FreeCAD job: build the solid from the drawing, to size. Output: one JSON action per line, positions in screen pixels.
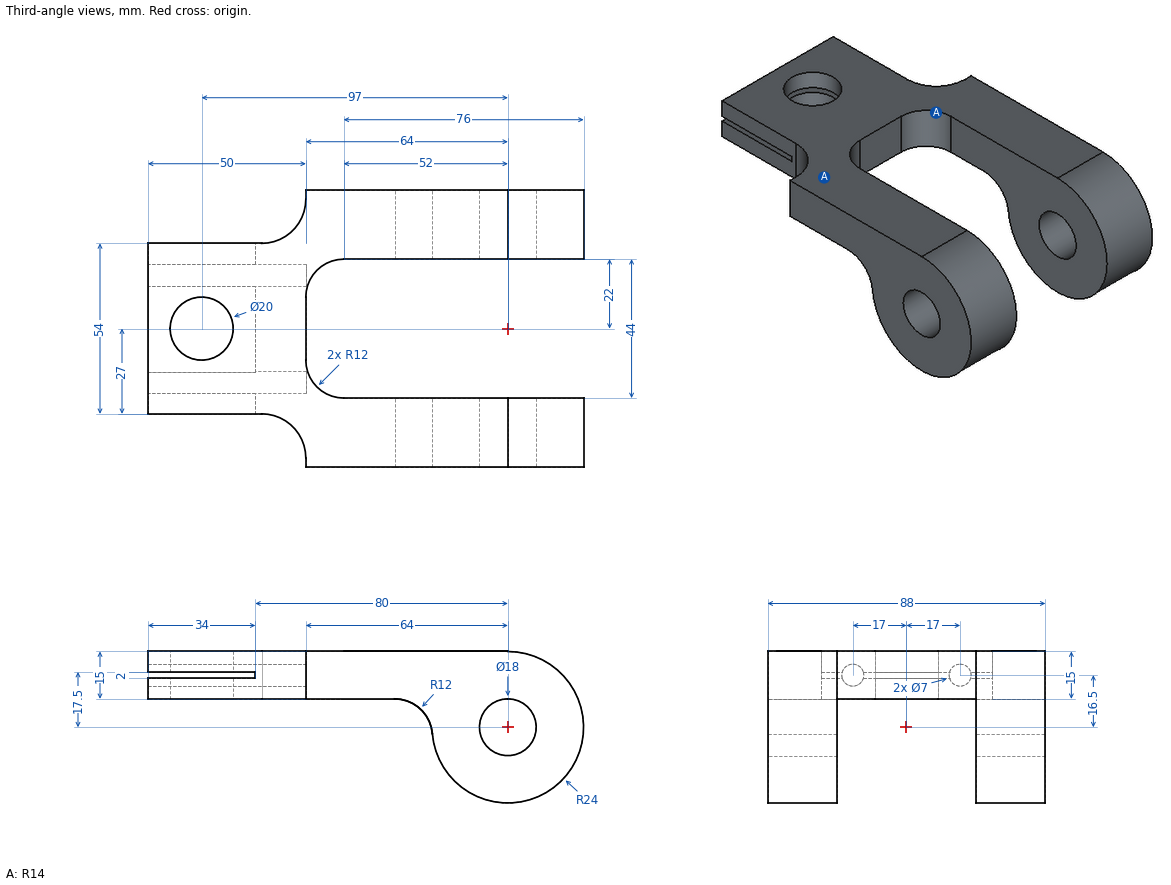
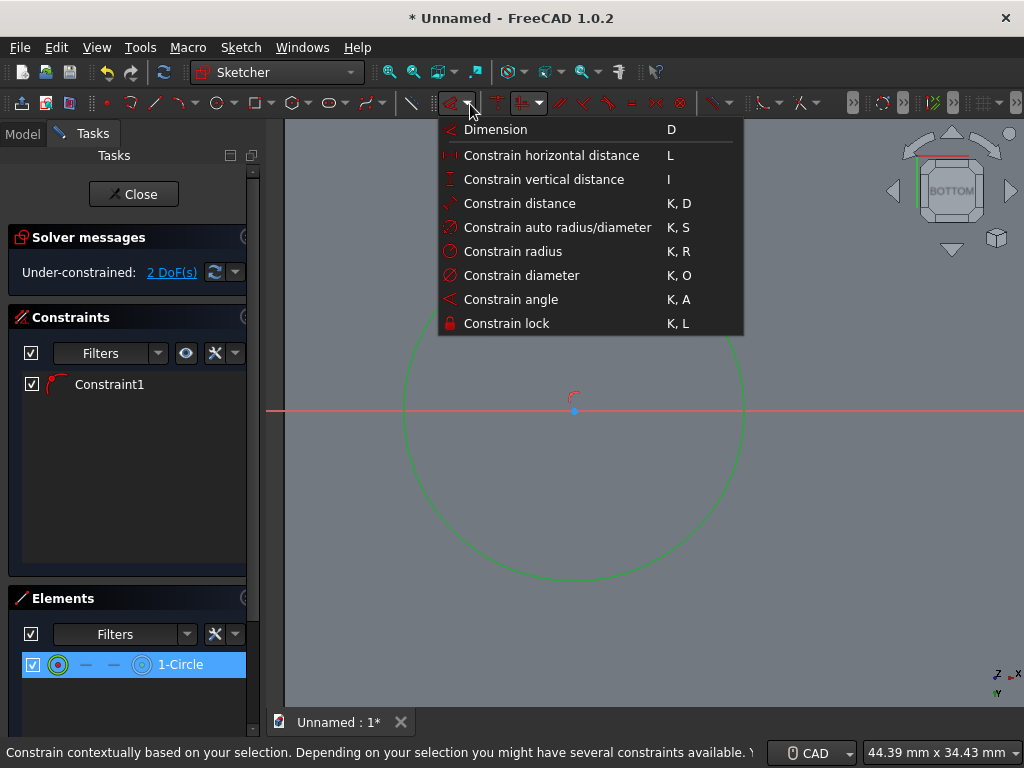
{"action": "left_click", "coordinate": [591, 275]}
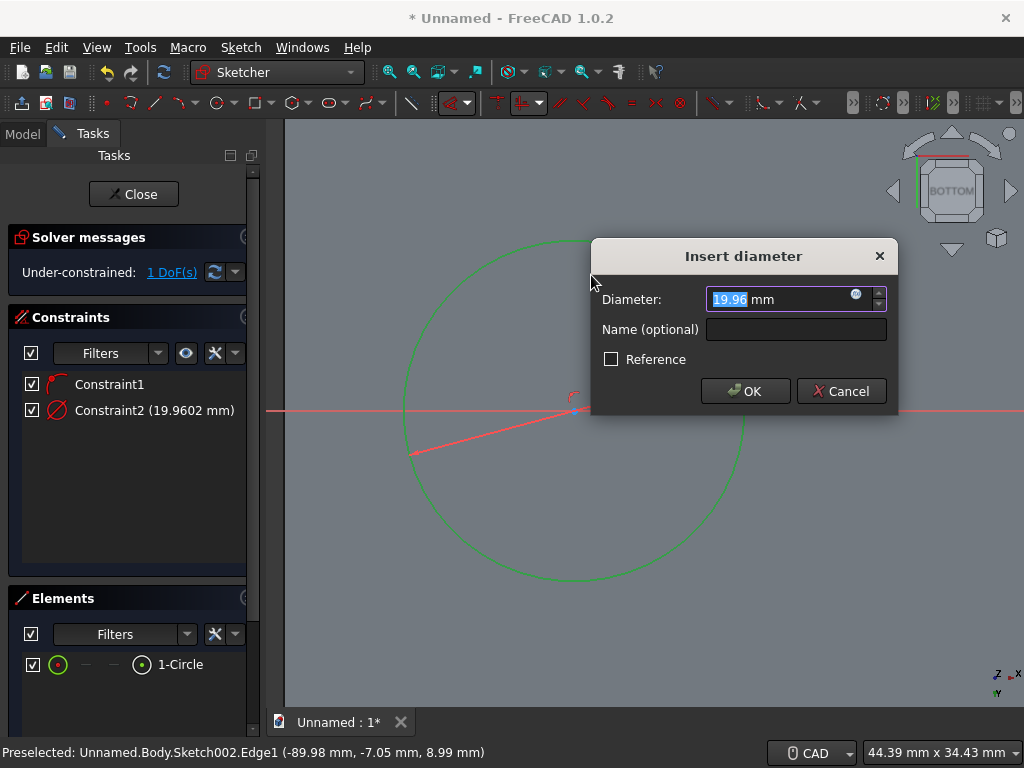
{"action": "type", "text": "20"}
{"action": "key", "text": "Return"}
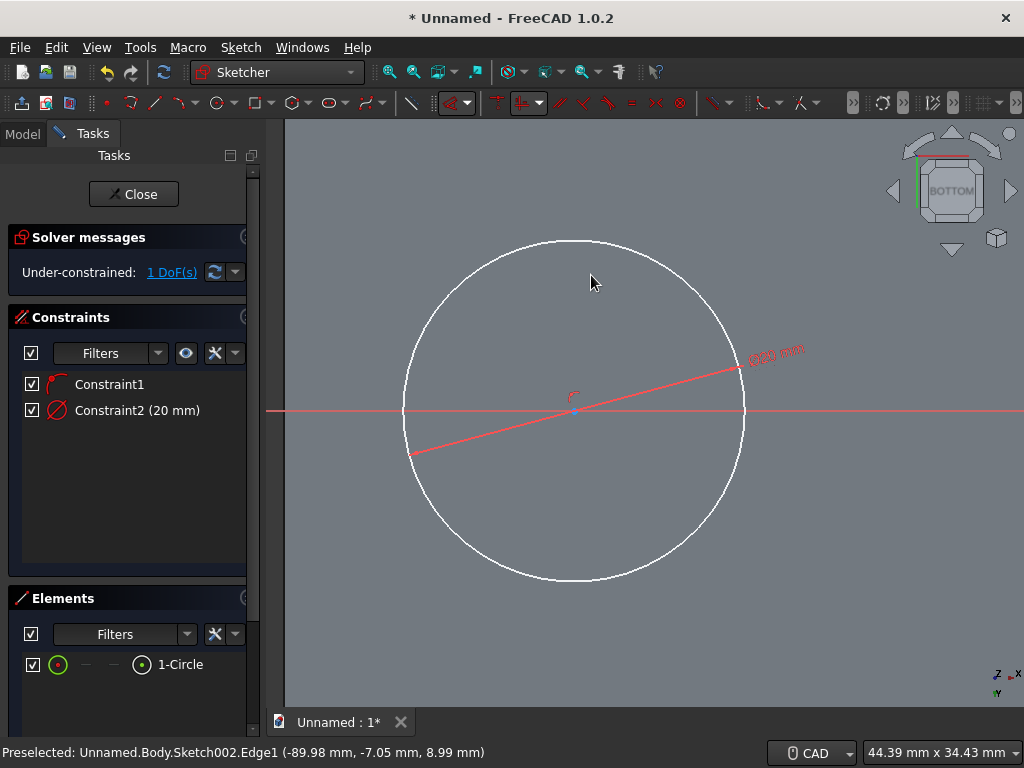
{"action": "left_click", "coordinate": [574, 411]}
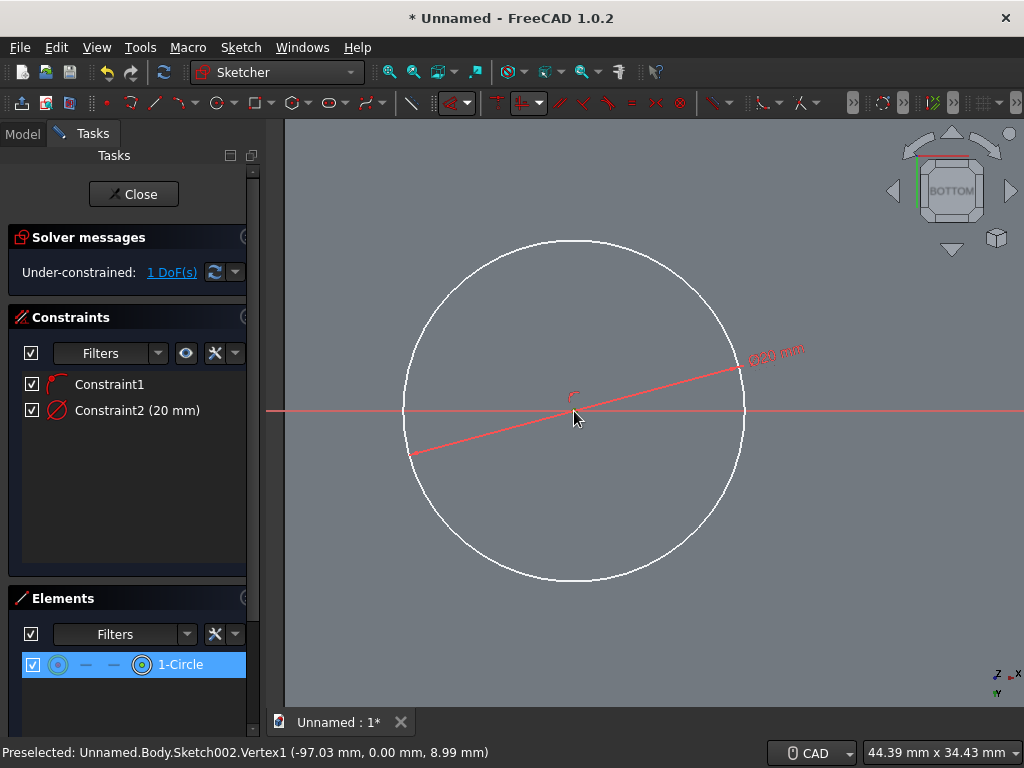
{"action": "key", "text": "l"}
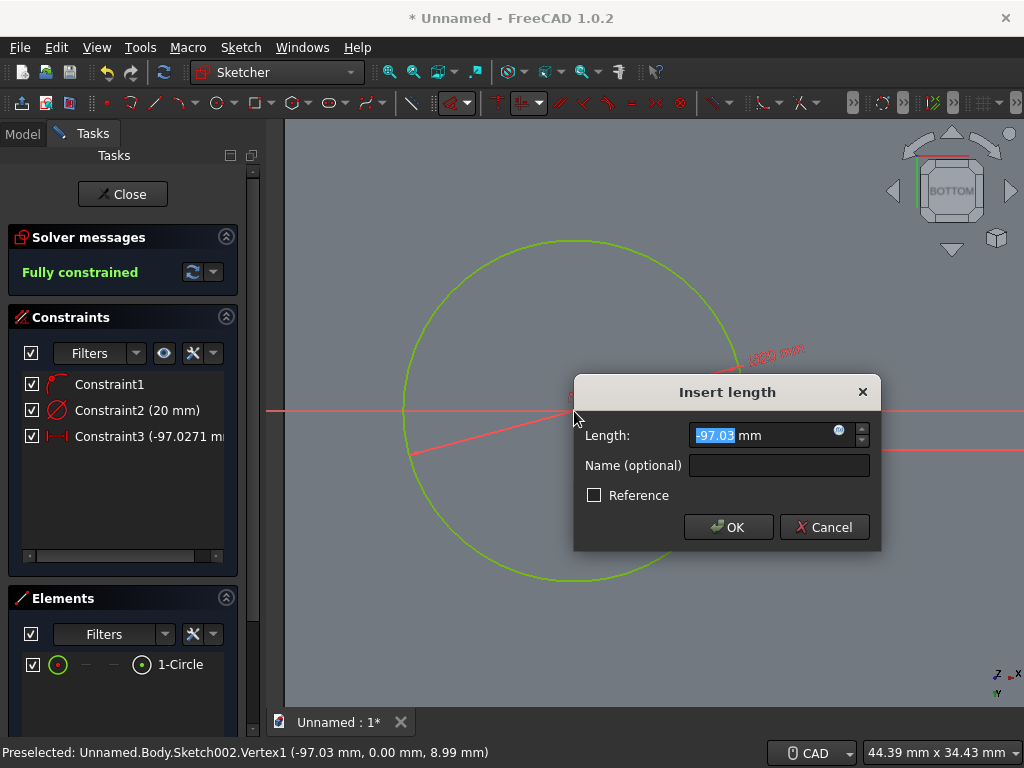
{"action": "type", "text": "-97"}
{"action": "key", "text": "Return"}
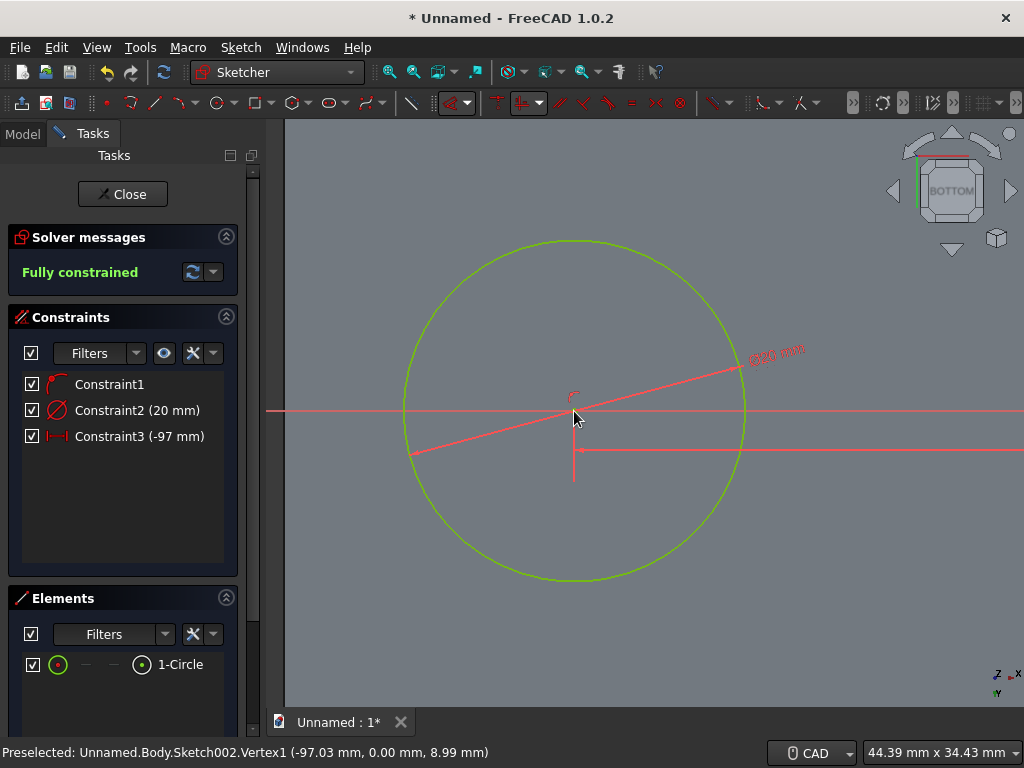
{"action": "left_click", "coordinate": [123, 194]}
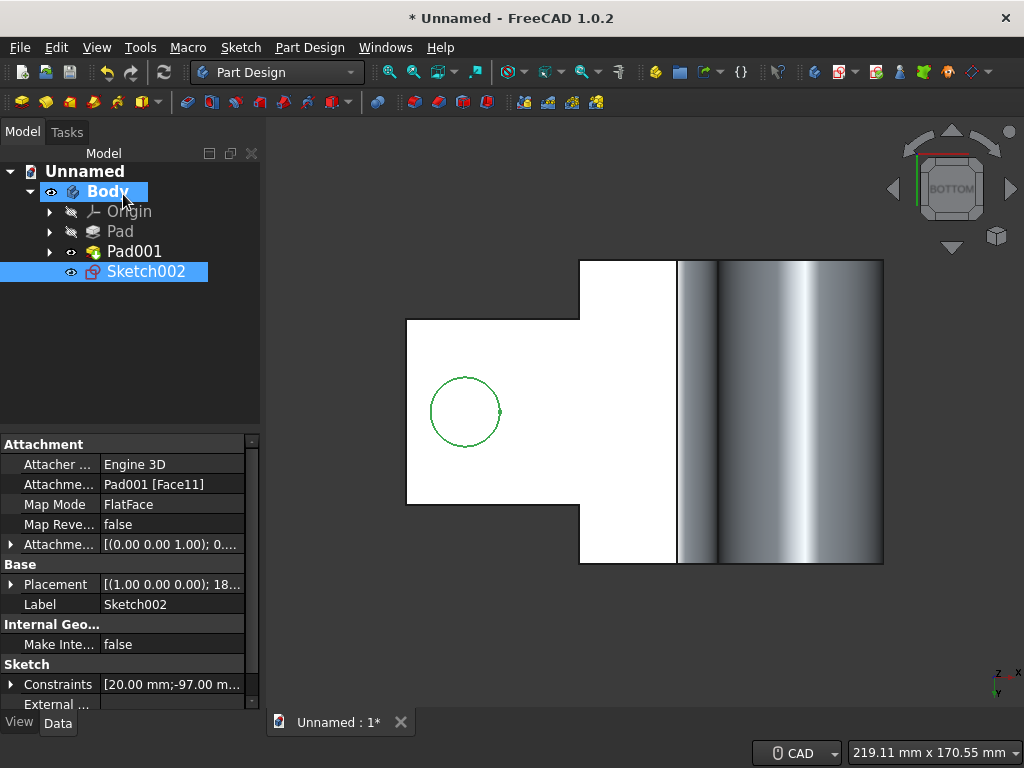
{"action": "left_click", "coordinate": [188, 102]}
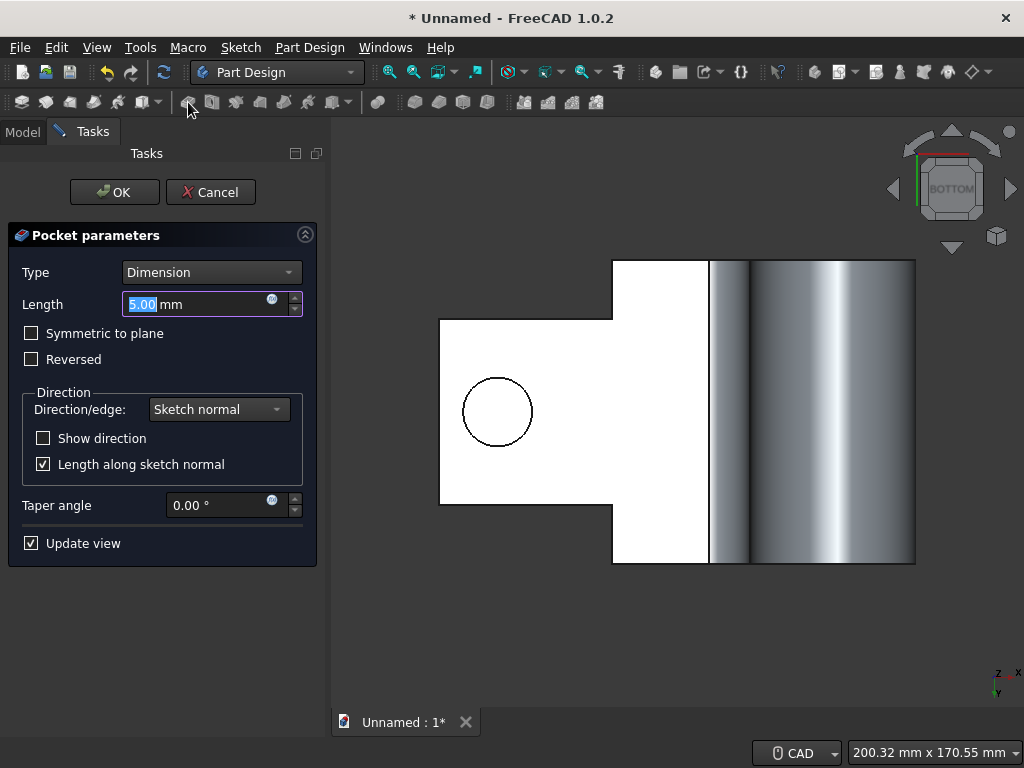
{"action": "left_click", "coordinate": [212, 272]}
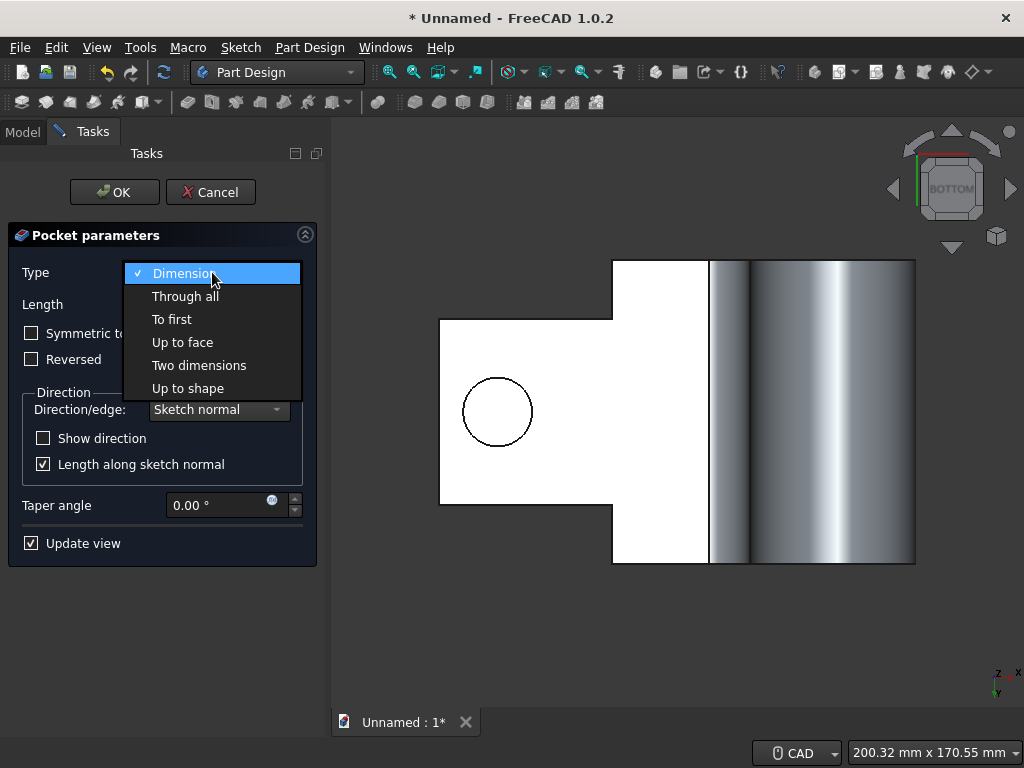
{"action": "left_click", "coordinate": [212, 320]}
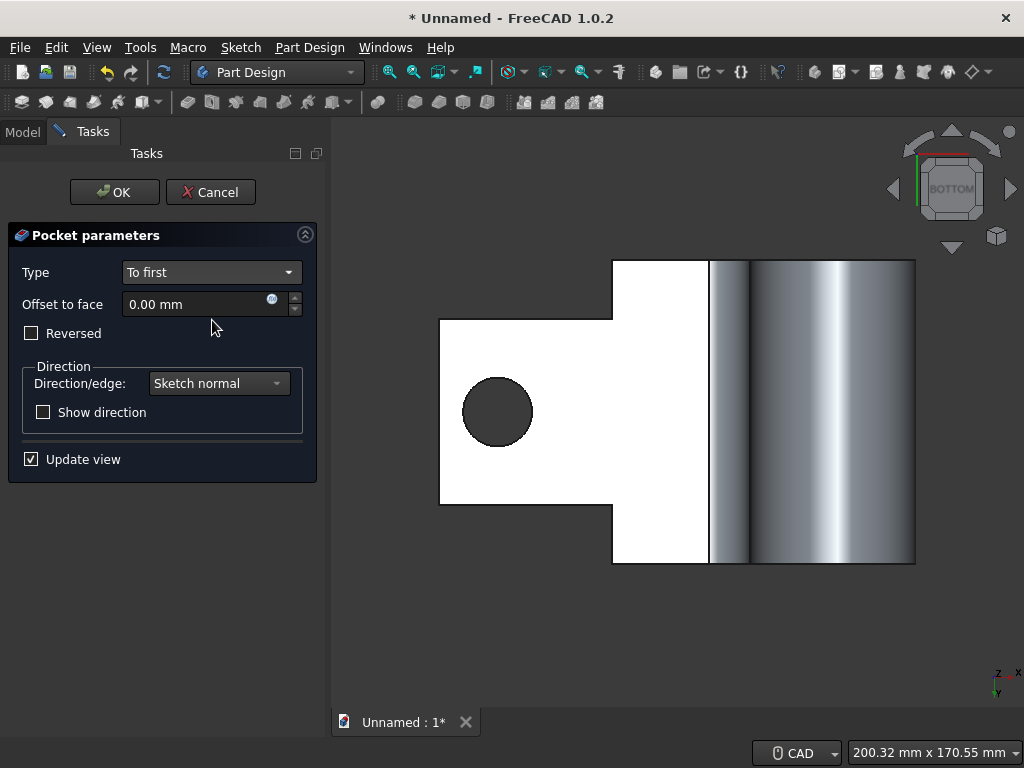
{"action": "left_click", "coordinate": [115, 192]}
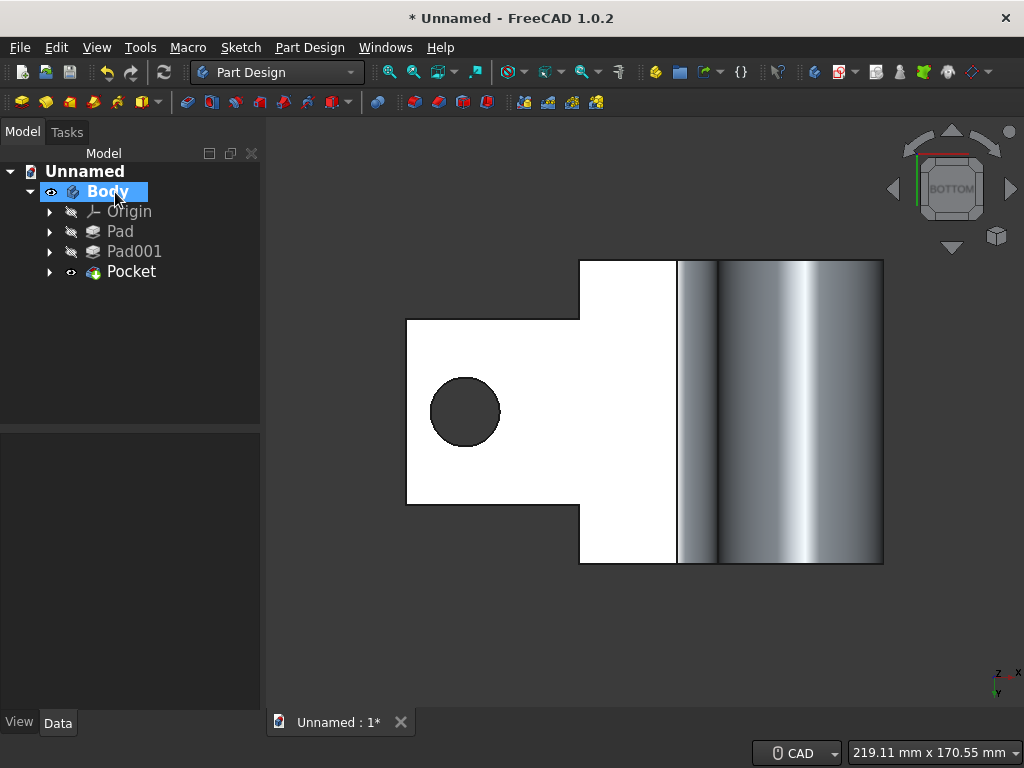
{"action": "key", "text": "0"}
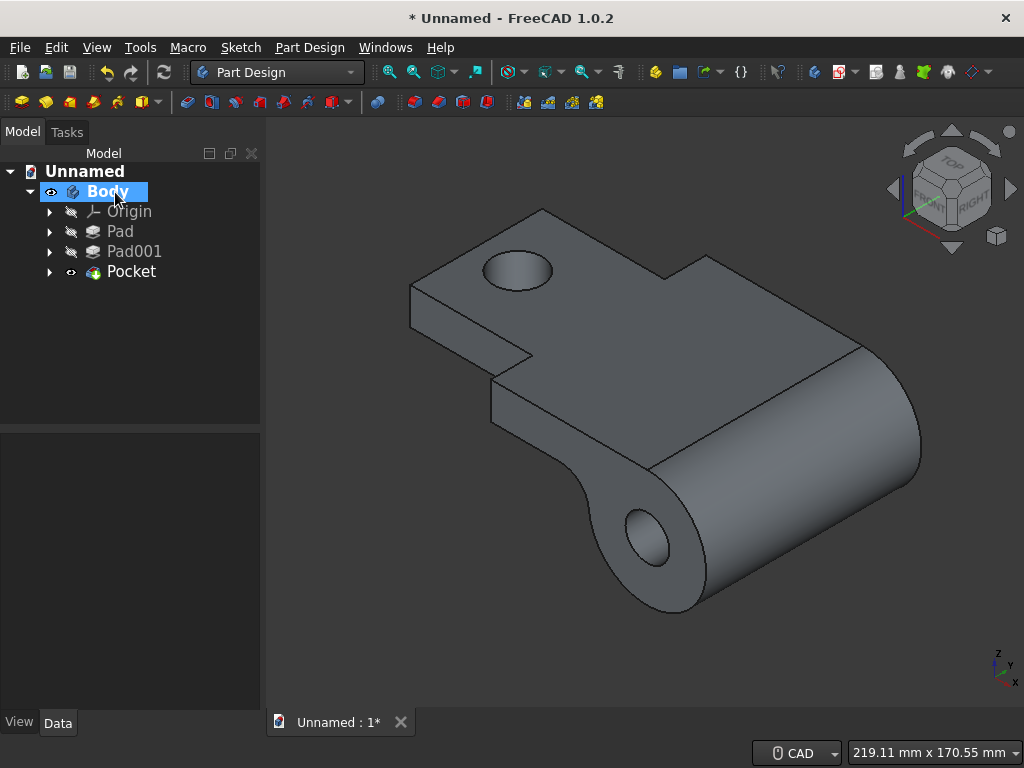
{"action": "left_click", "coordinate": [489, 351]}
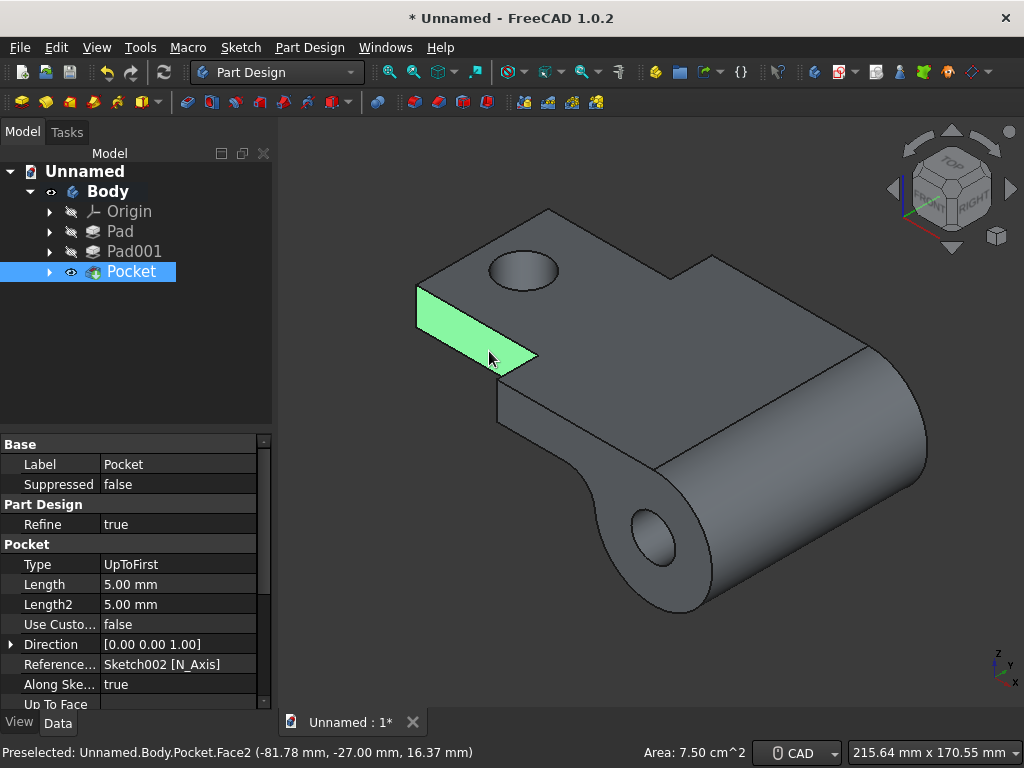
{"action": "left_click", "coordinate": [840, 72]}